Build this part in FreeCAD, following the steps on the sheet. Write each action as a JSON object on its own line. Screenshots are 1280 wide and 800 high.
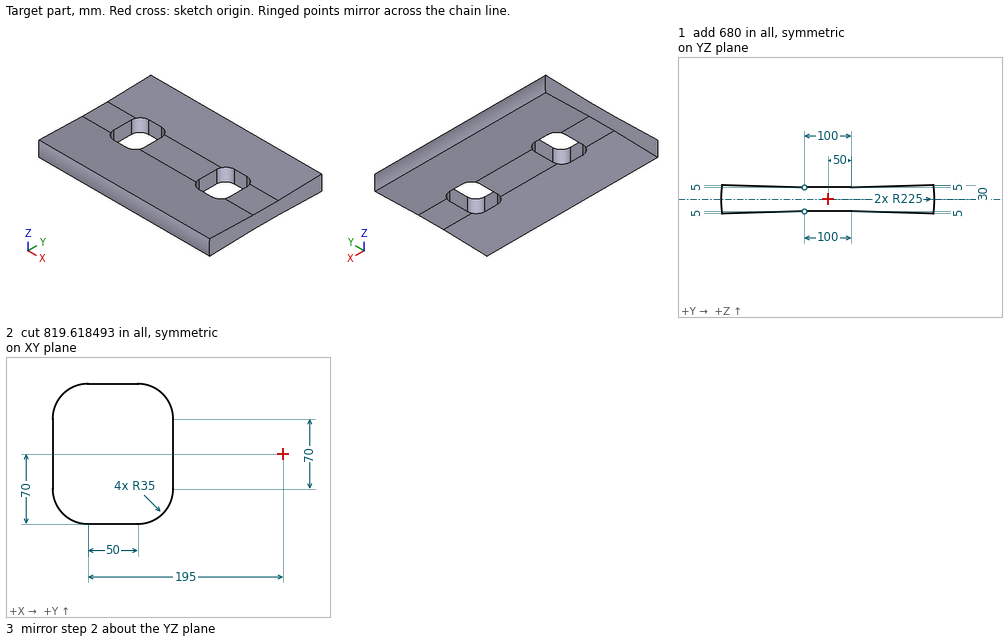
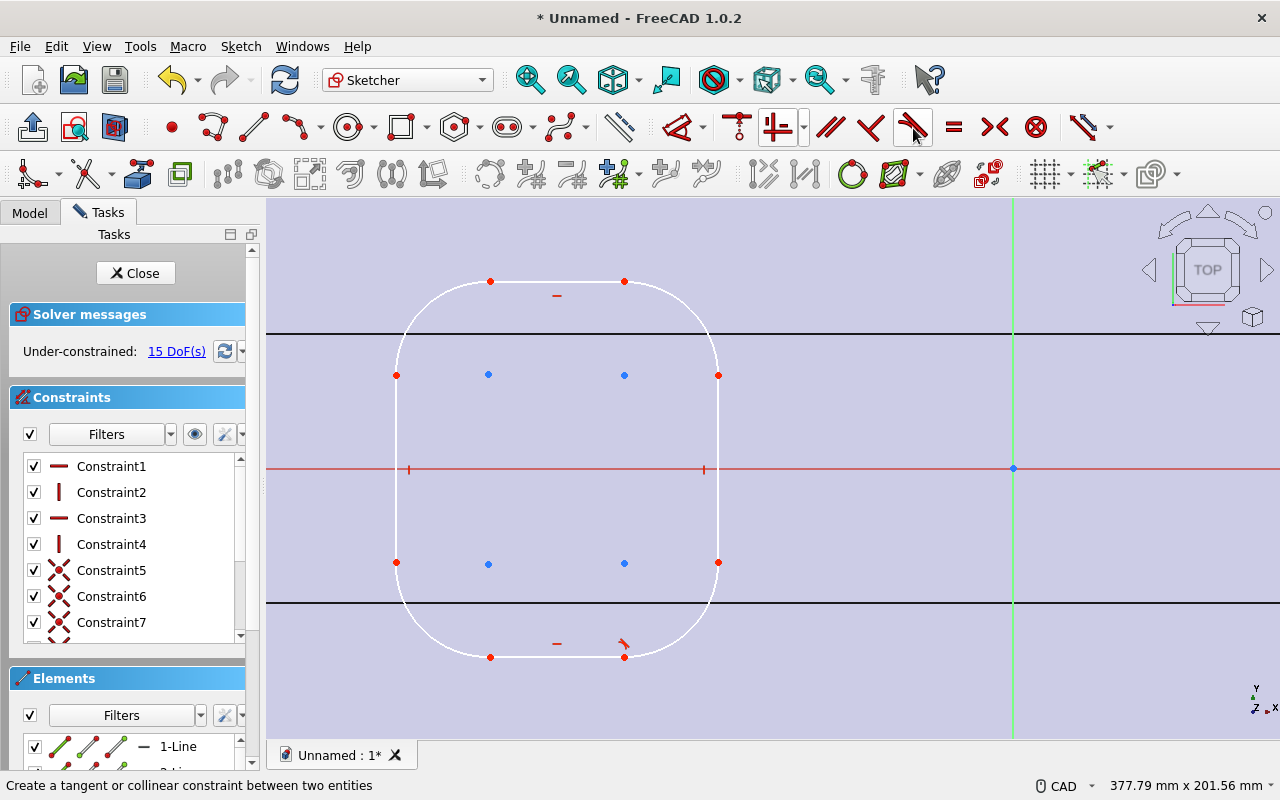
{"action": "left_click", "coordinate": [530, 657]}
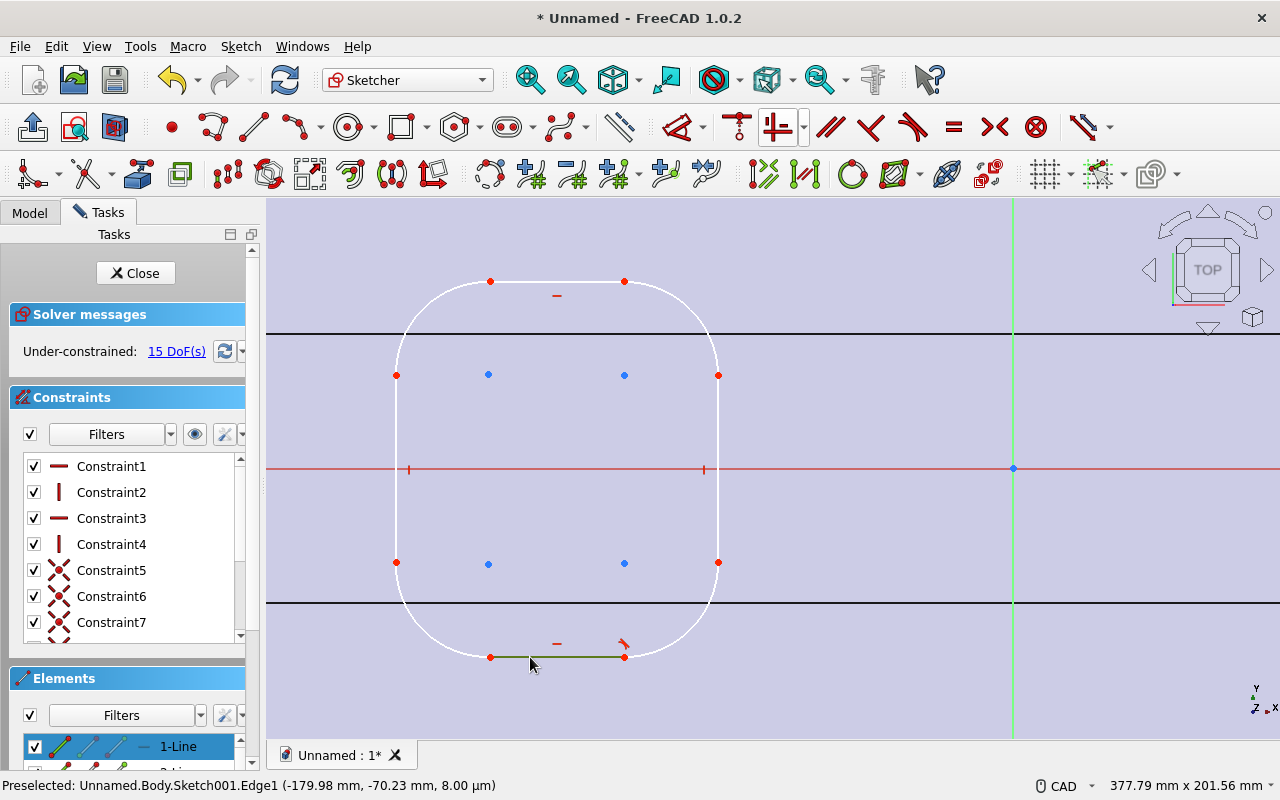
{"action": "left_click", "coordinate": [406, 606]}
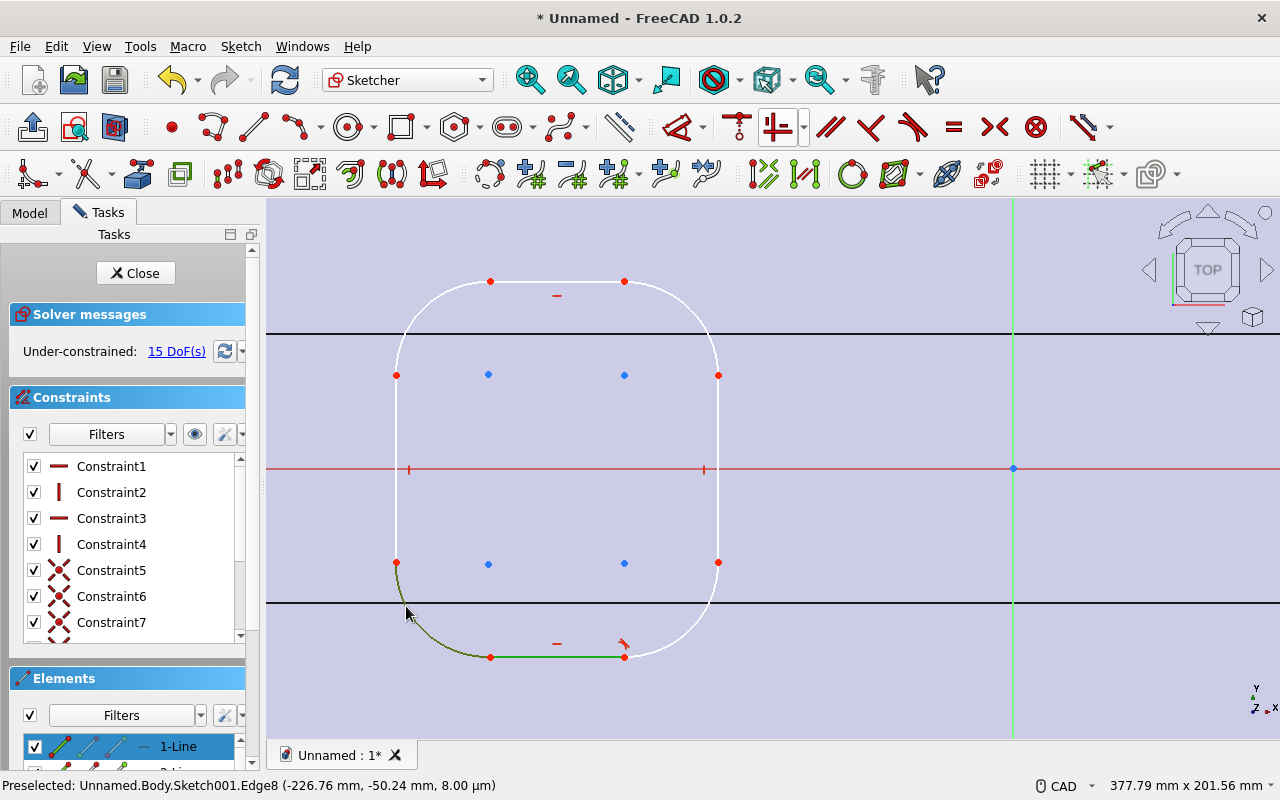
{"action": "key", "text": "t"}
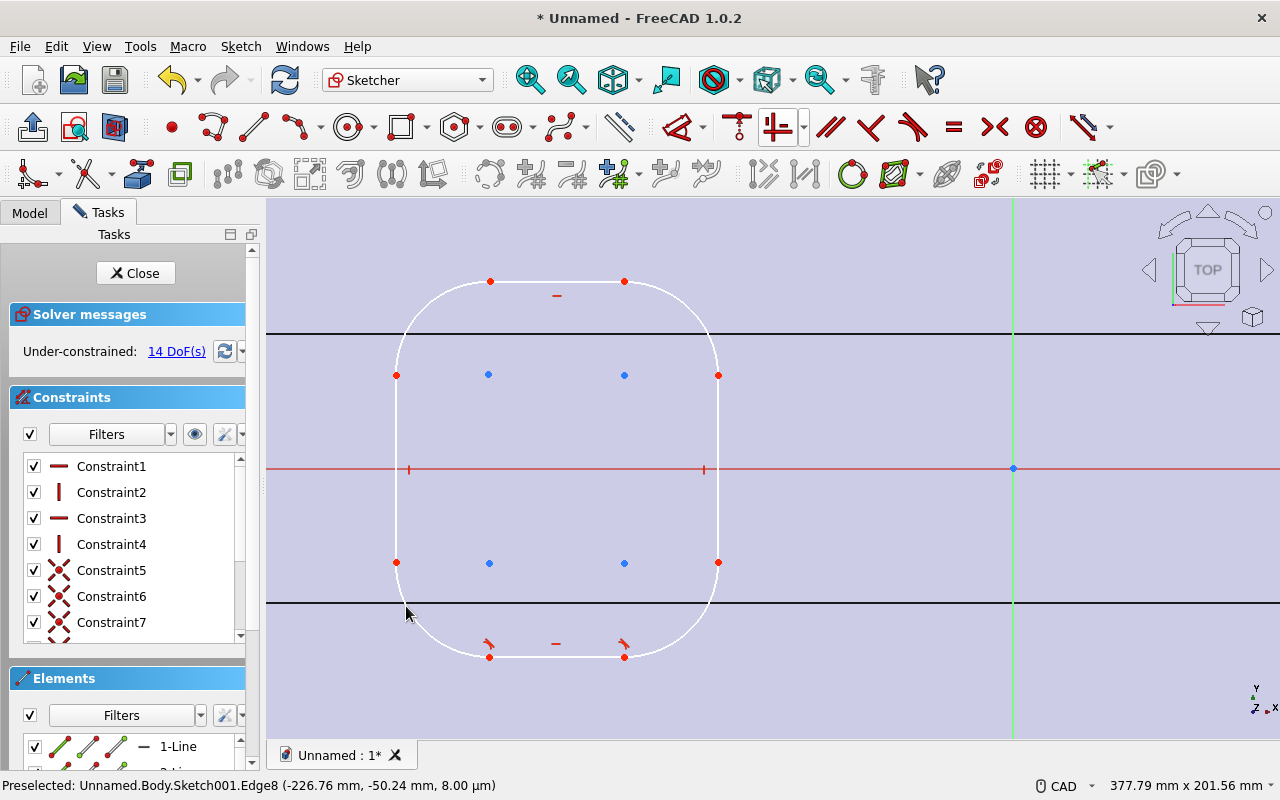
{"action": "left_click", "coordinate": [718, 507]}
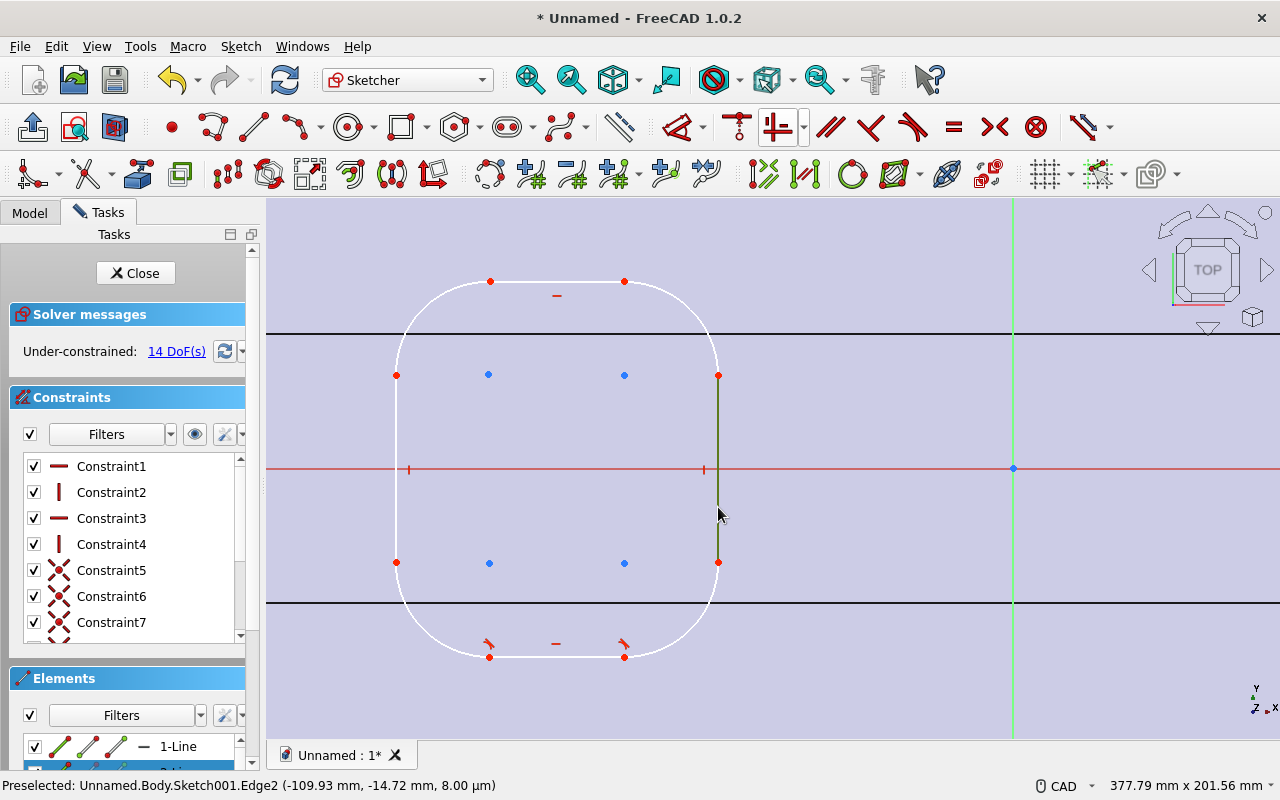
{"action": "left_click", "coordinate": [667, 647]}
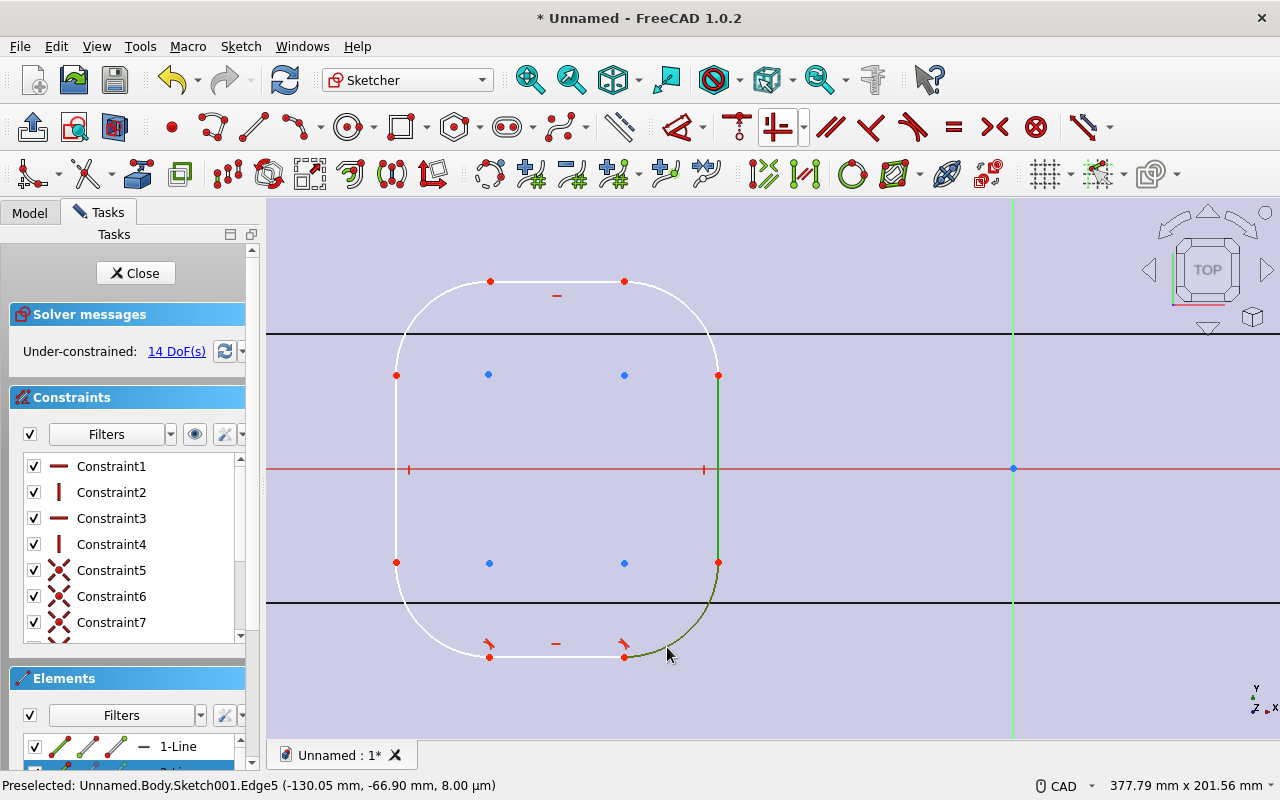
{"action": "key", "text": "t"}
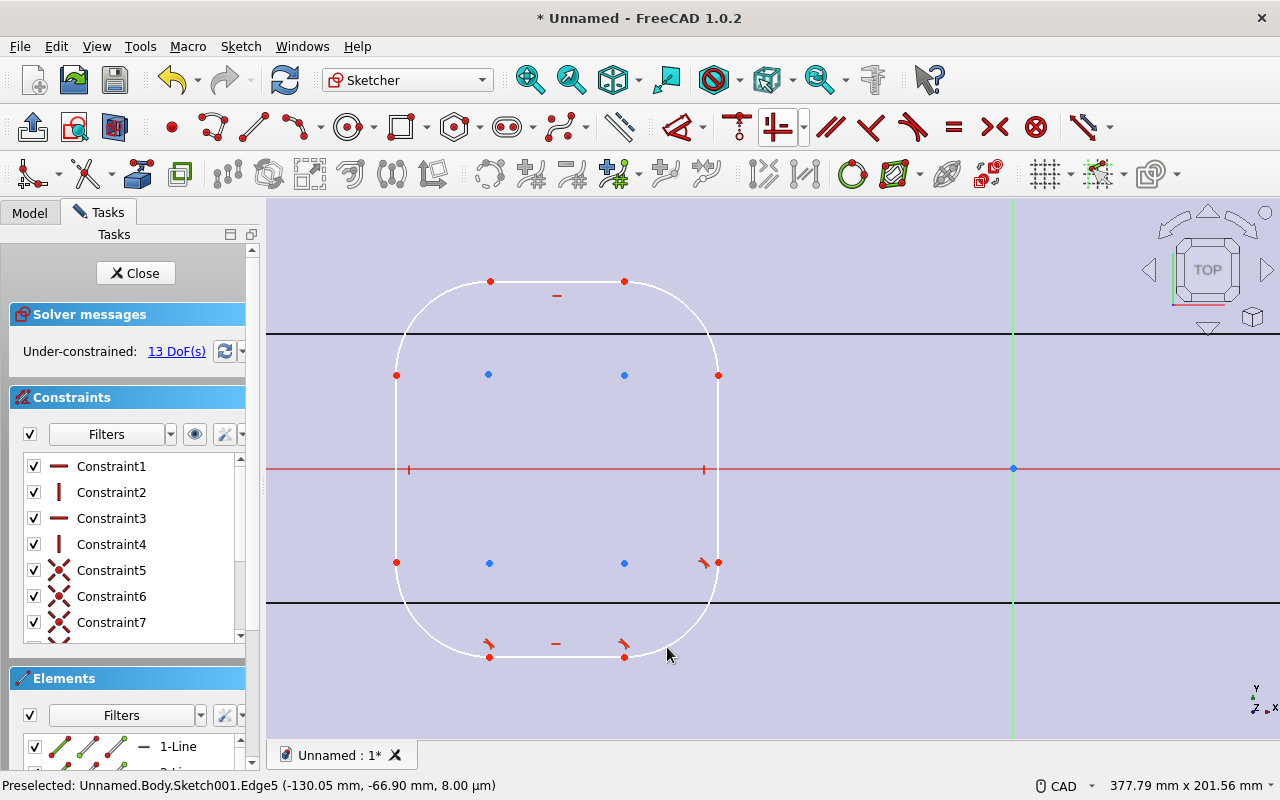
{"action": "left_click", "coordinate": [718, 507]}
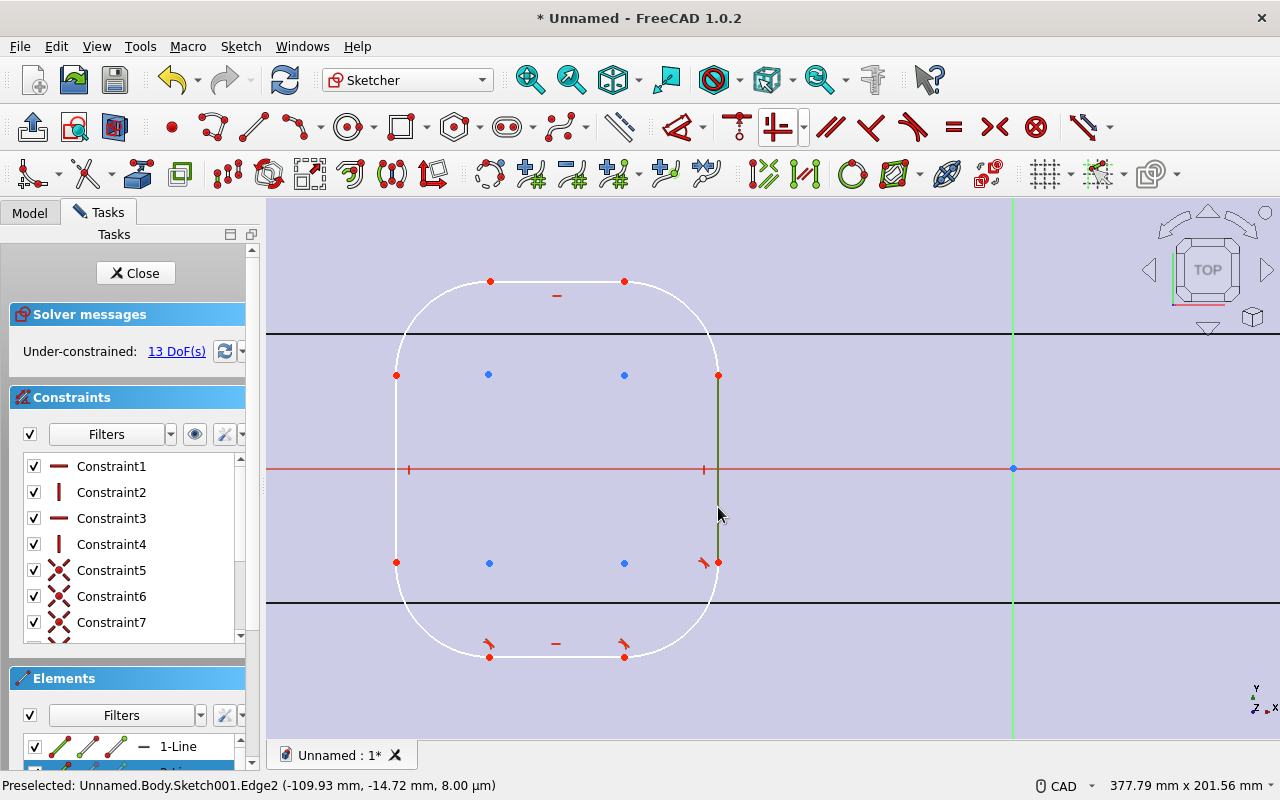
{"action": "left_click", "coordinate": [708, 333]}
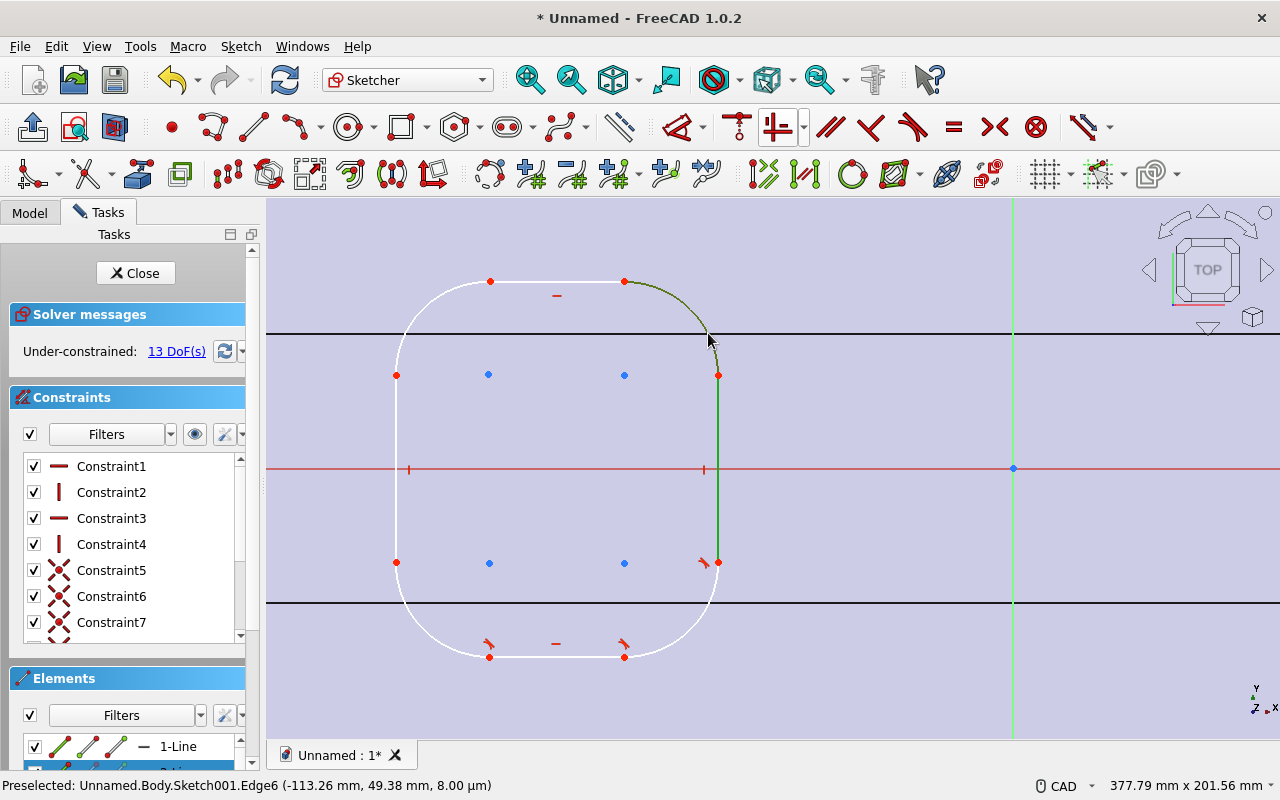
{"action": "left_click", "coordinate": [913, 128]}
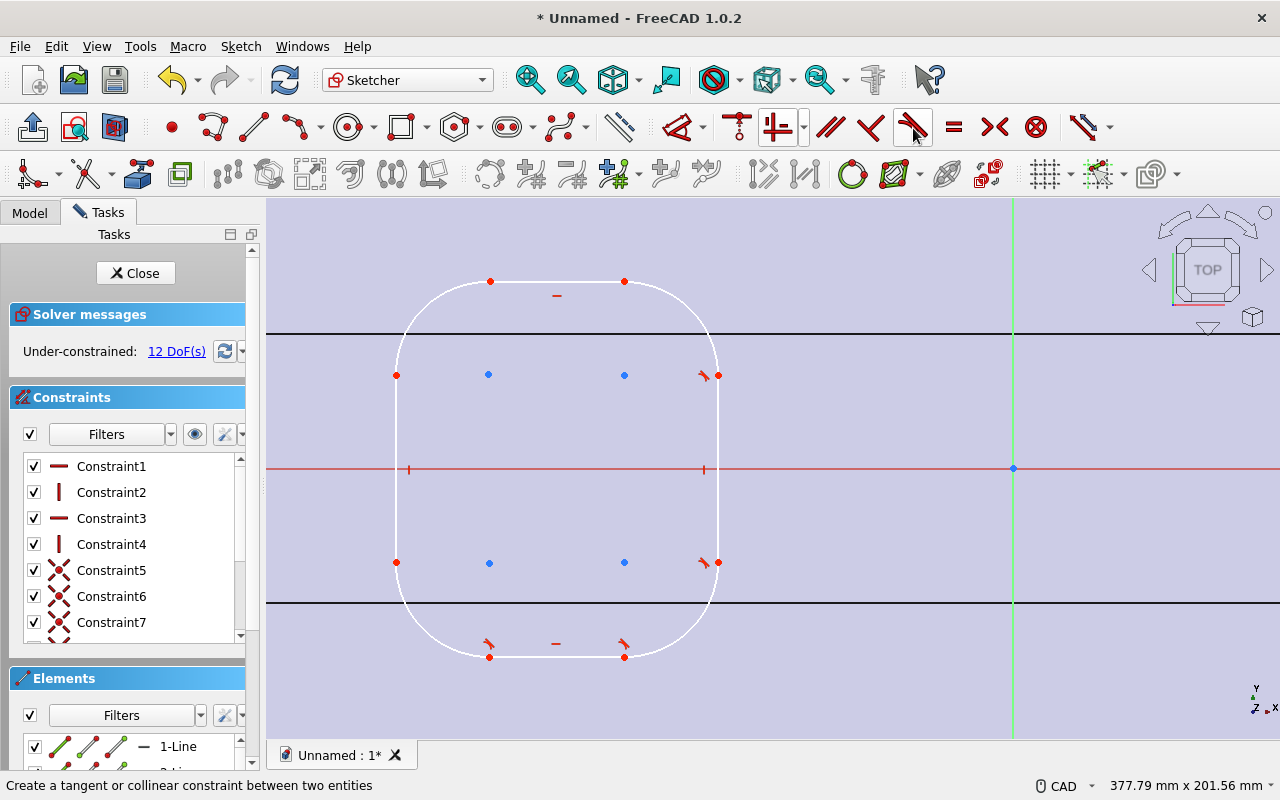
{"action": "left_click", "coordinate": [584, 282]}